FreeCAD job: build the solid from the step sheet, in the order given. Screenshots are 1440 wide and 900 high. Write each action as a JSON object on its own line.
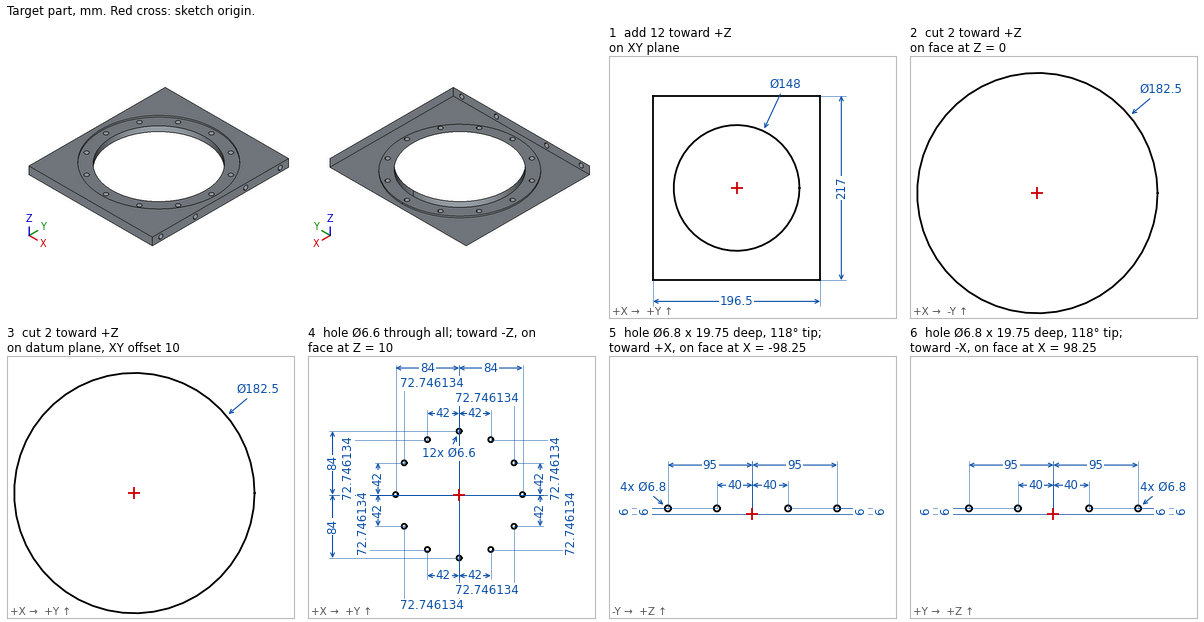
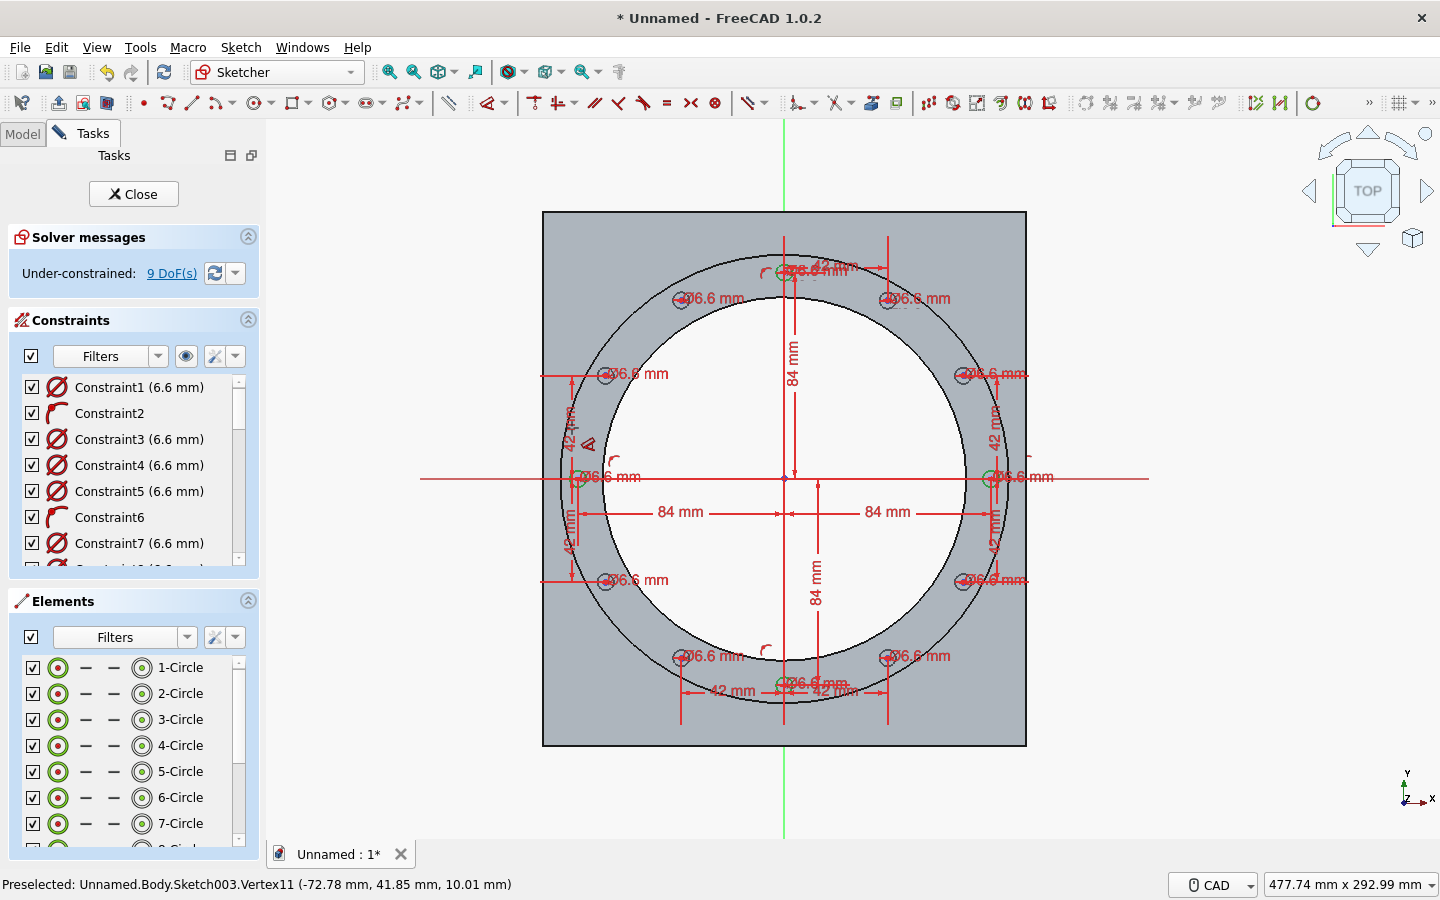
{"action": "left_click", "coordinate": [681, 300]}
{"action": "left_click", "coordinate": [733, 266]}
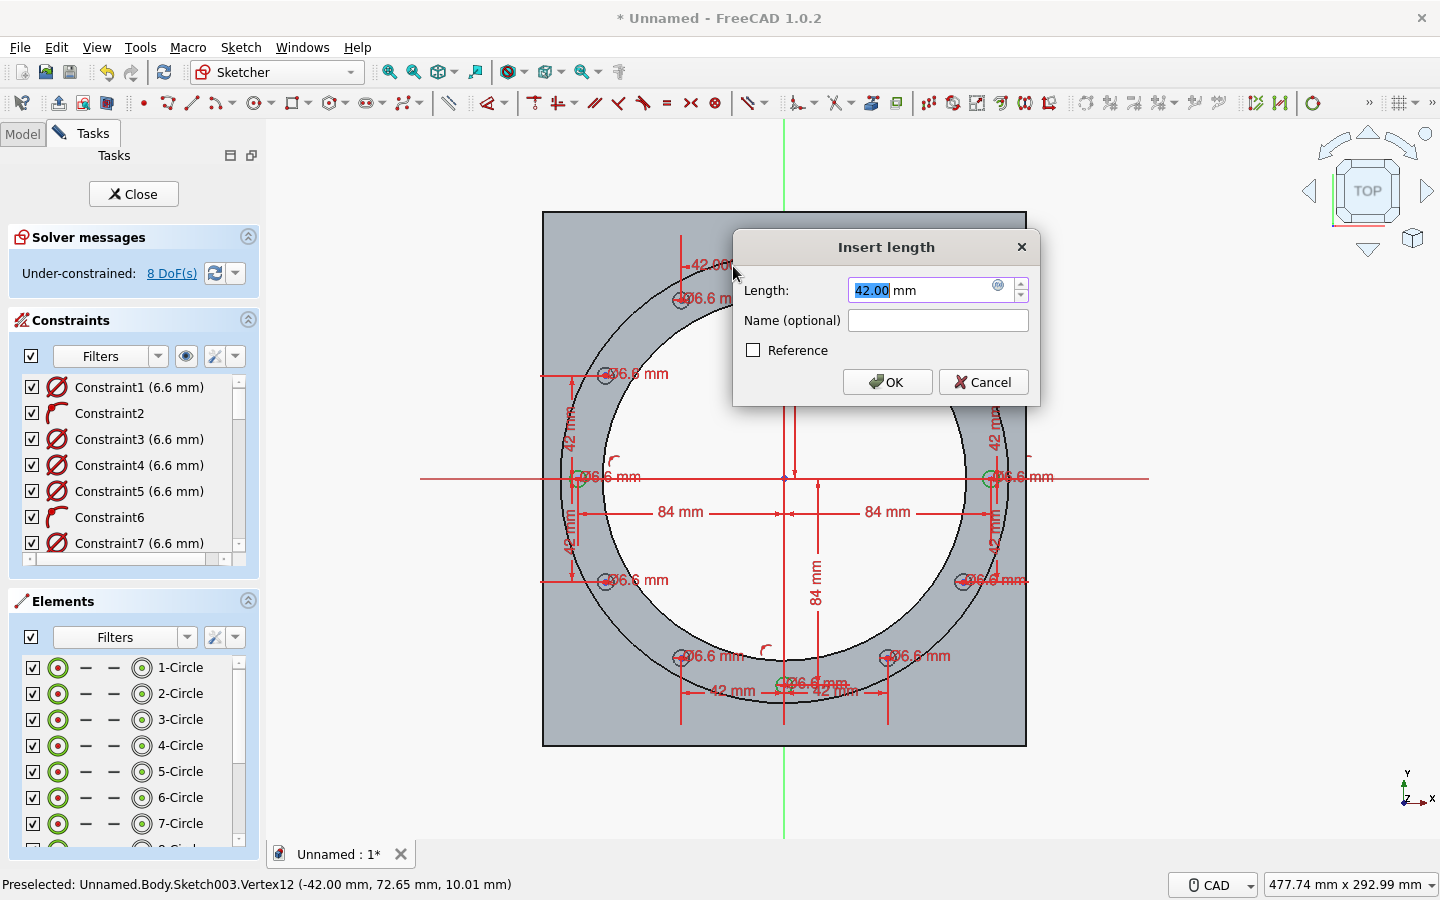
{"action": "type", "text": "42"}
{"action": "key", "text": "Return"}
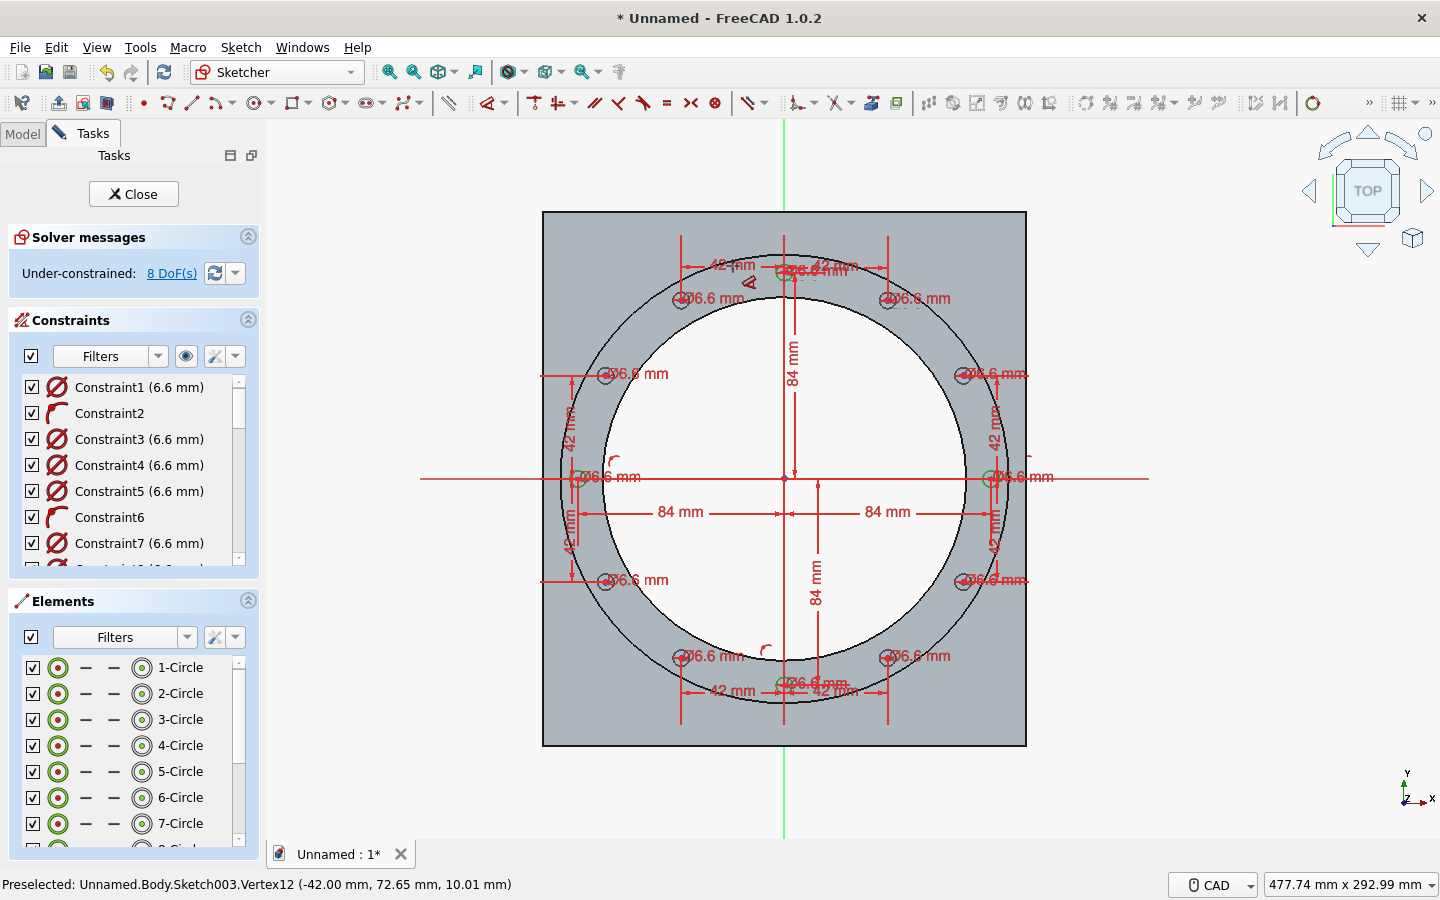
{"action": "left_click", "coordinate": [888, 301]}
{"action": "left_click", "coordinate": [922, 390]}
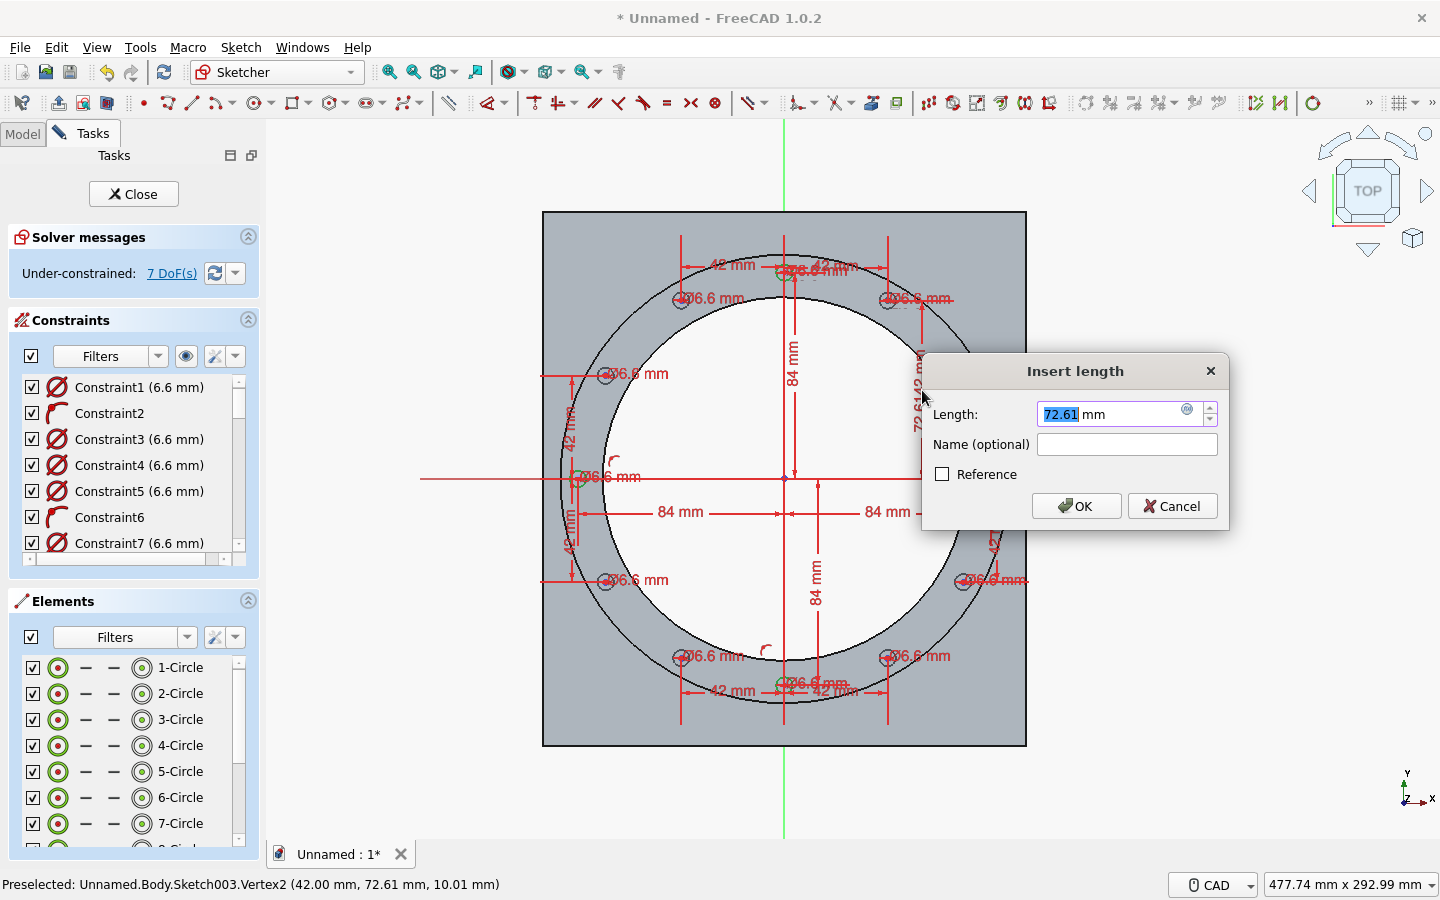
{"action": "type", "text": "72.746134"}
{"action": "key", "text": "Return"}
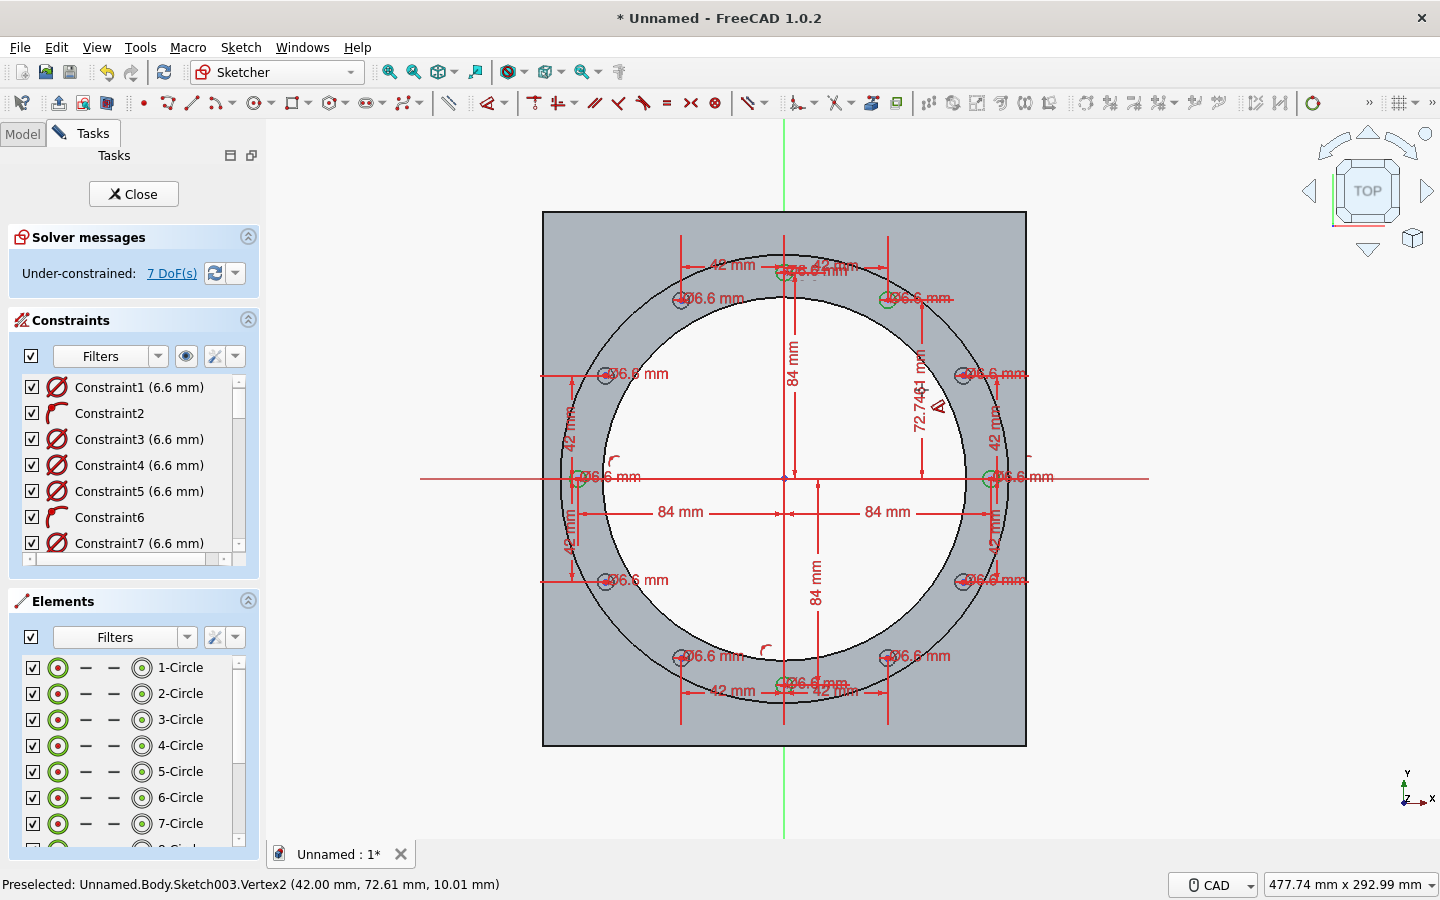
{"action": "left_click", "coordinate": [963, 376]}
{"action": "left_click", "coordinate": [874, 342]}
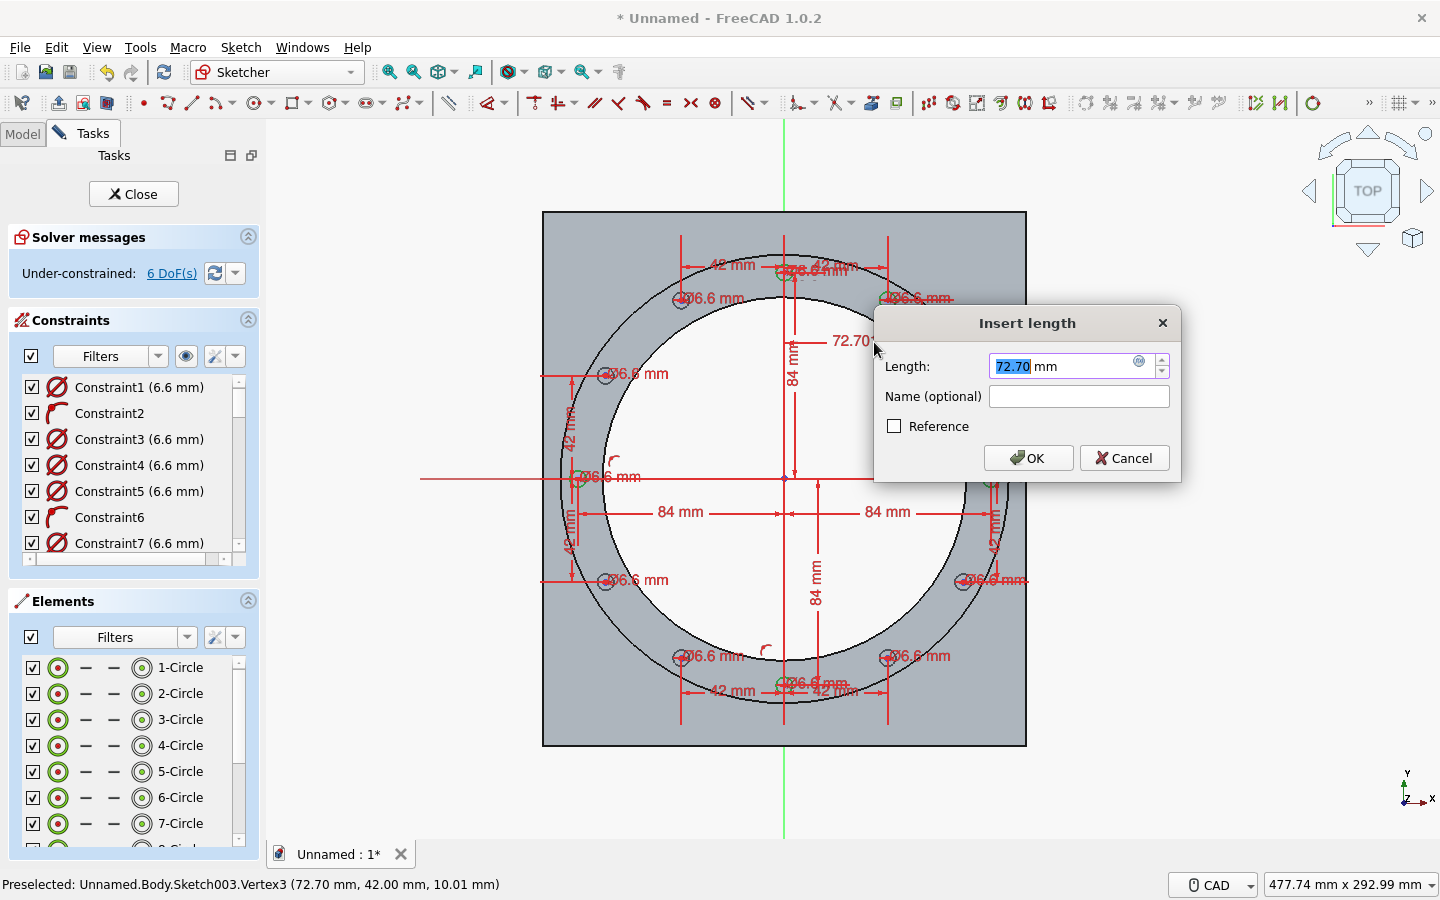
{"action": "type", "text": "72.746134"}
{"action": "key", "text": "Return"}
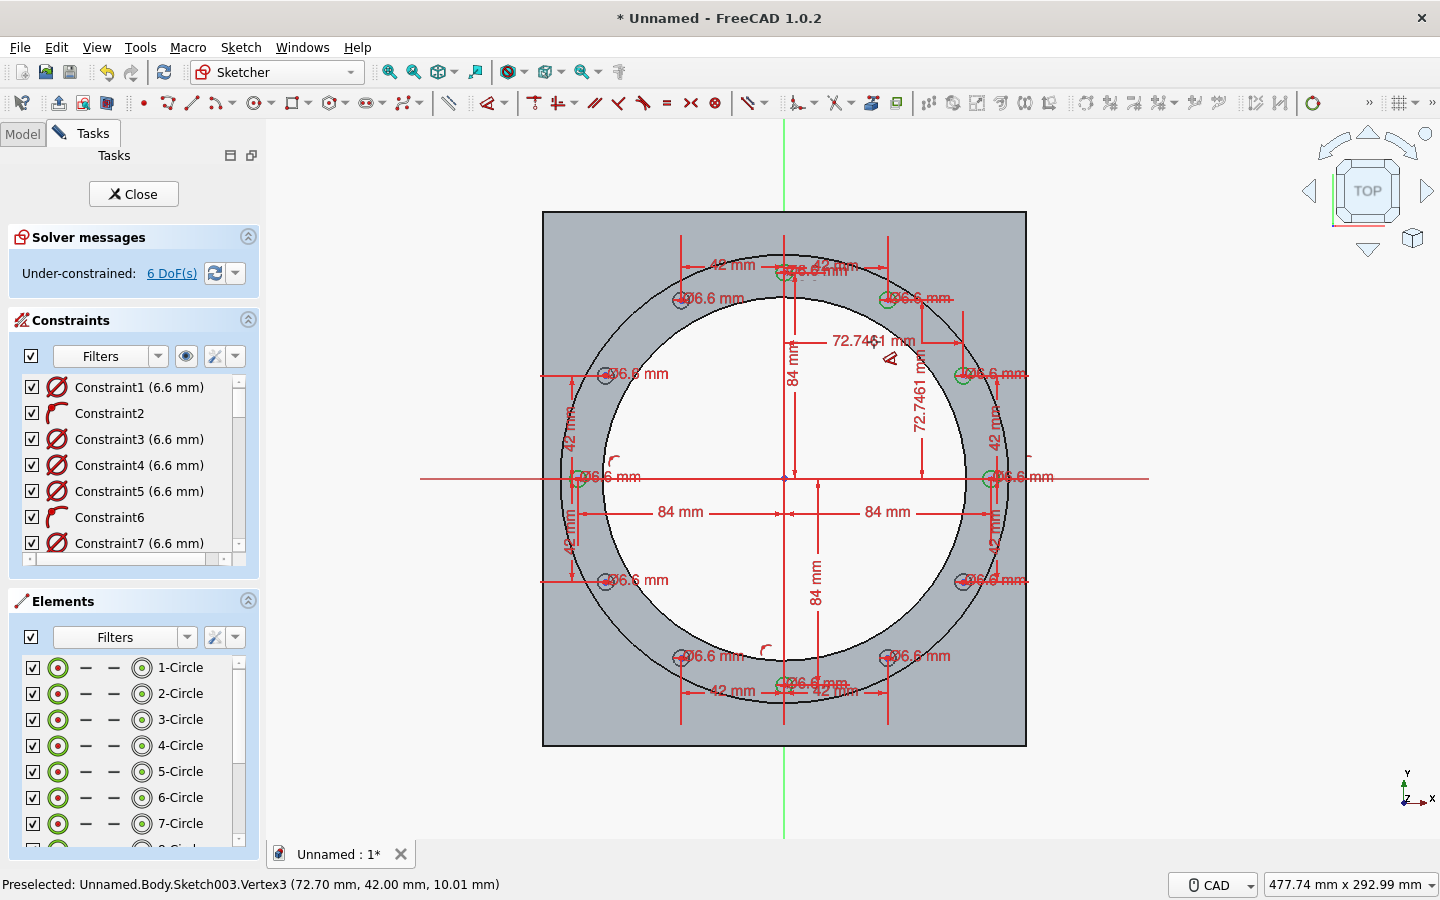
{"action": "left_click", "coordinate": [963, 582]}
{"action": "left_click", "coordinate": [874, 616]}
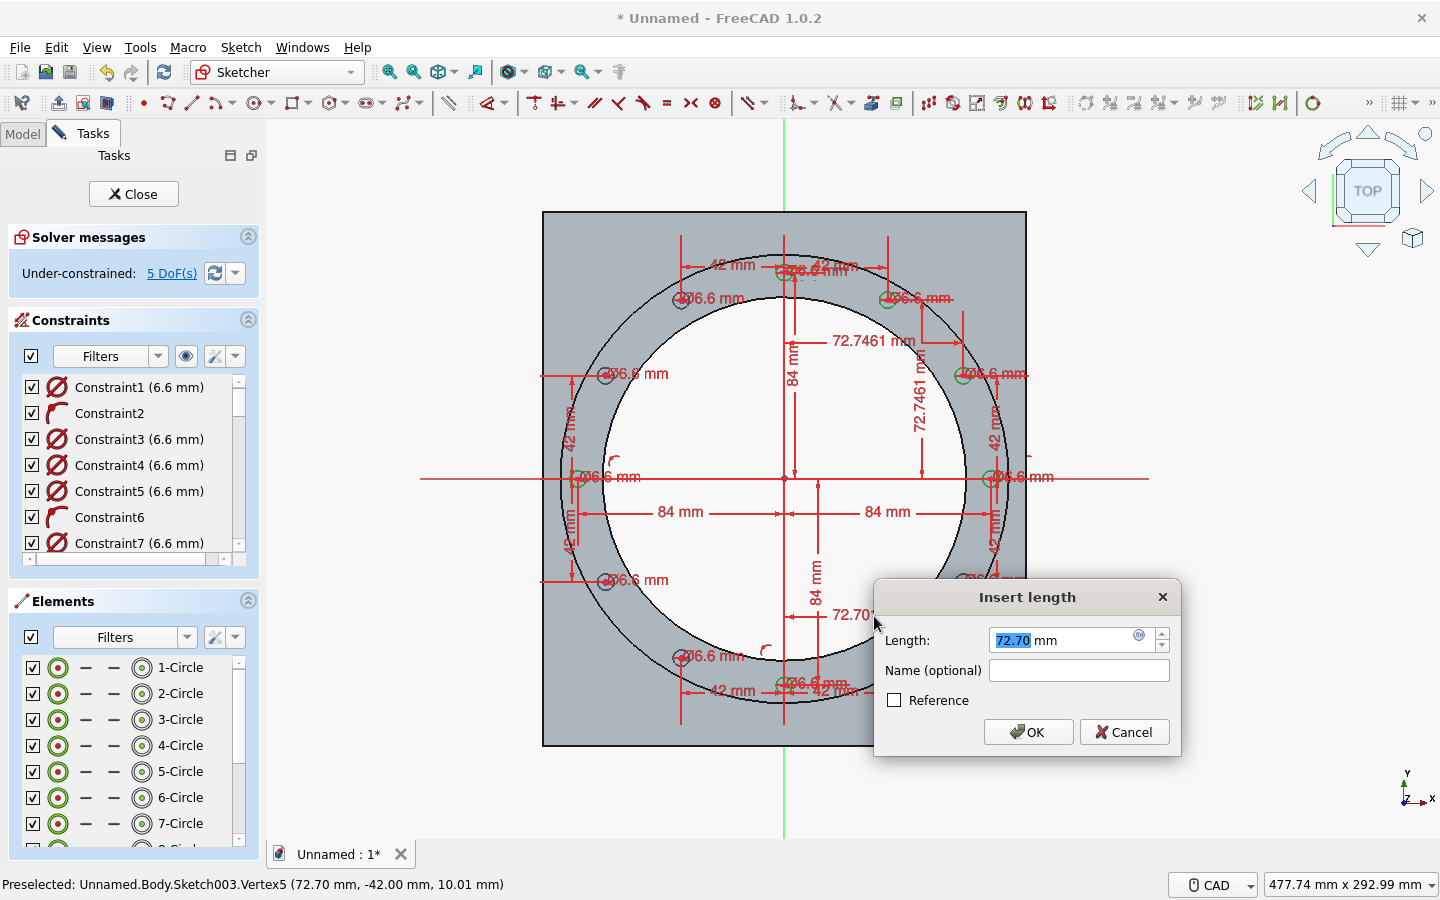
{"action": "type", "text": "72.746134"}
{"action": "key", "text": "Return"}